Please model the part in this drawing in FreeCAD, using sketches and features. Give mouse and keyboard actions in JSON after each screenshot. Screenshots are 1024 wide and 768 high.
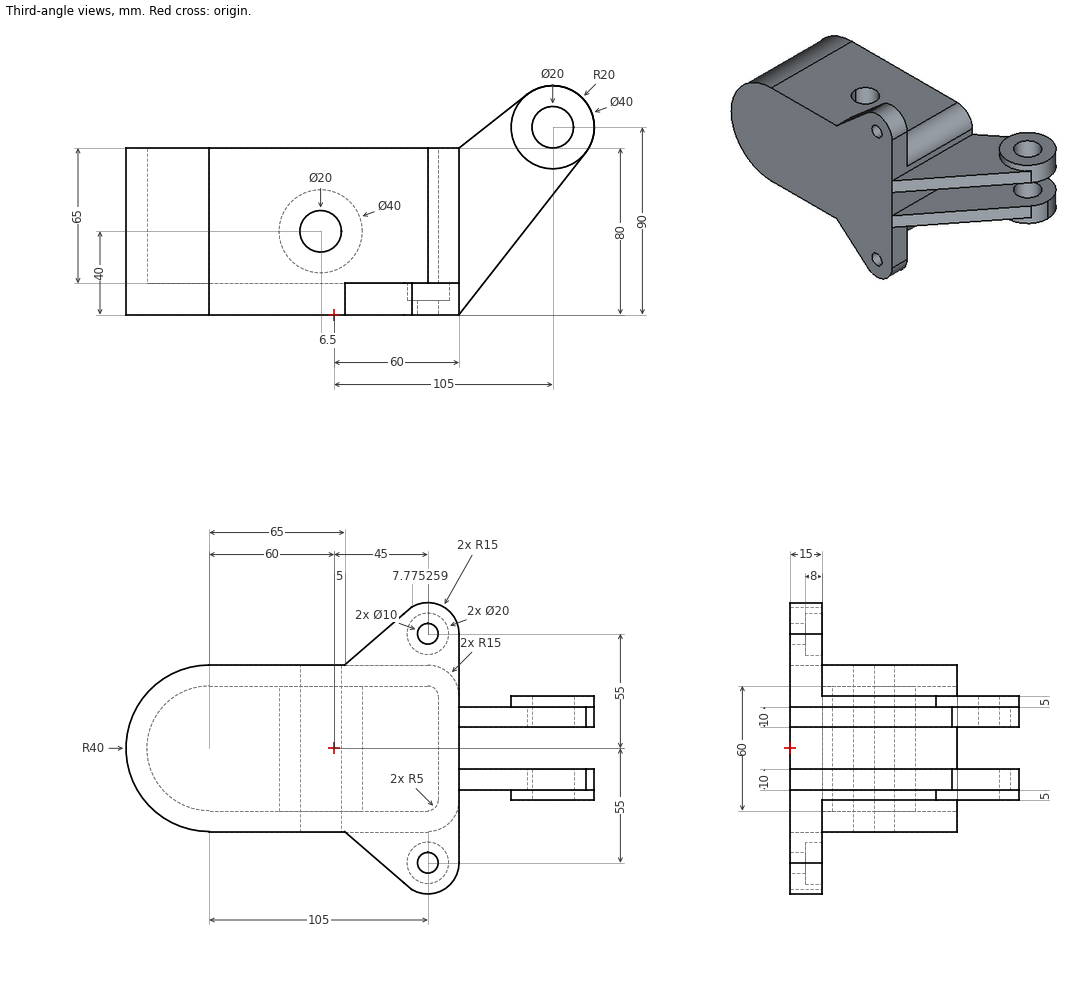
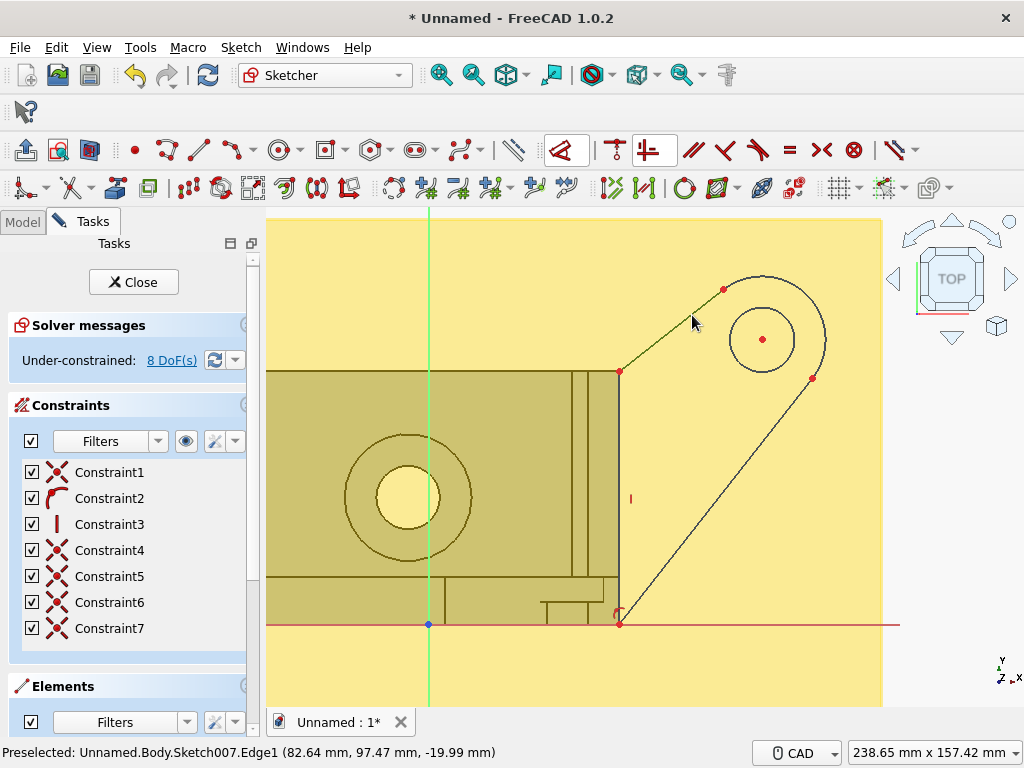
{"action": "left_click", "coordinate": [824, 327]}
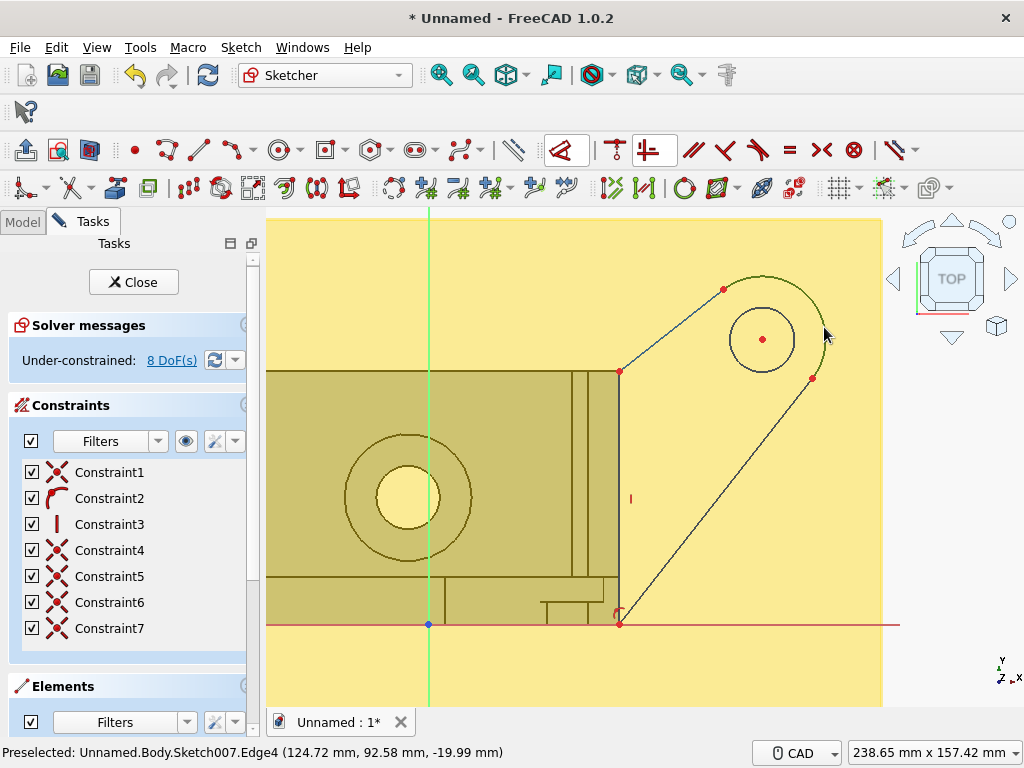
{"action": "left_click", "coordinate": [758, 150]}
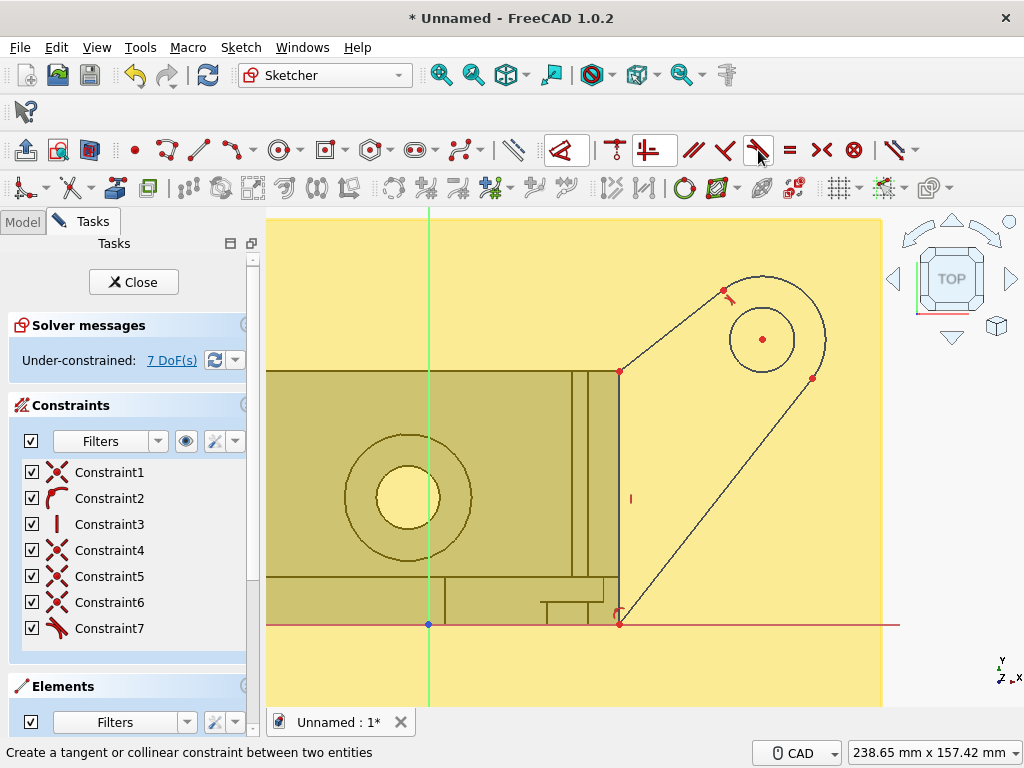
{"action": "left_click", "coordinate": [677, 551]}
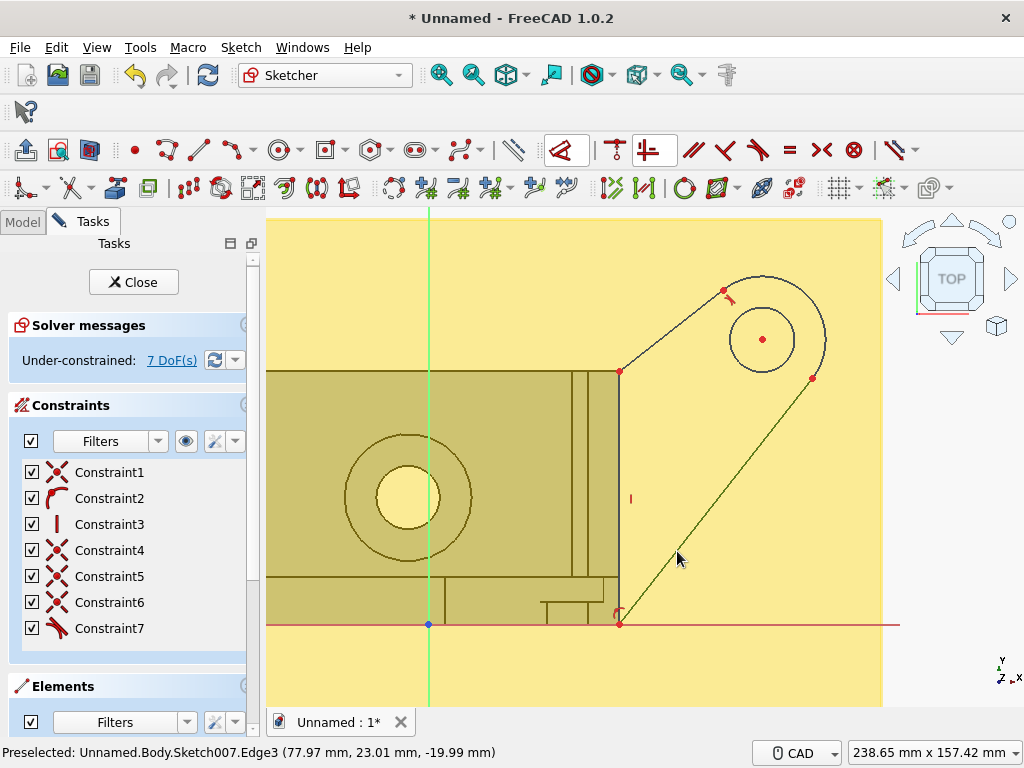
{"action": "left_click", "coordinate": [824, 327]}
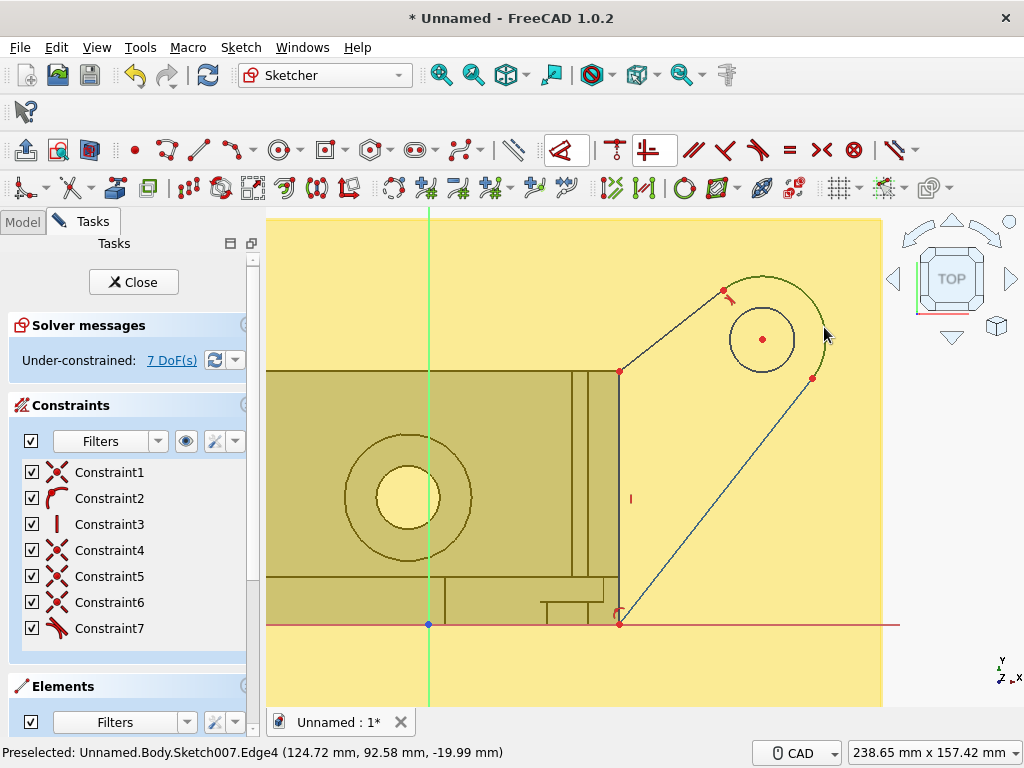
{"action": "left_click", "coordinate": [758, 150]}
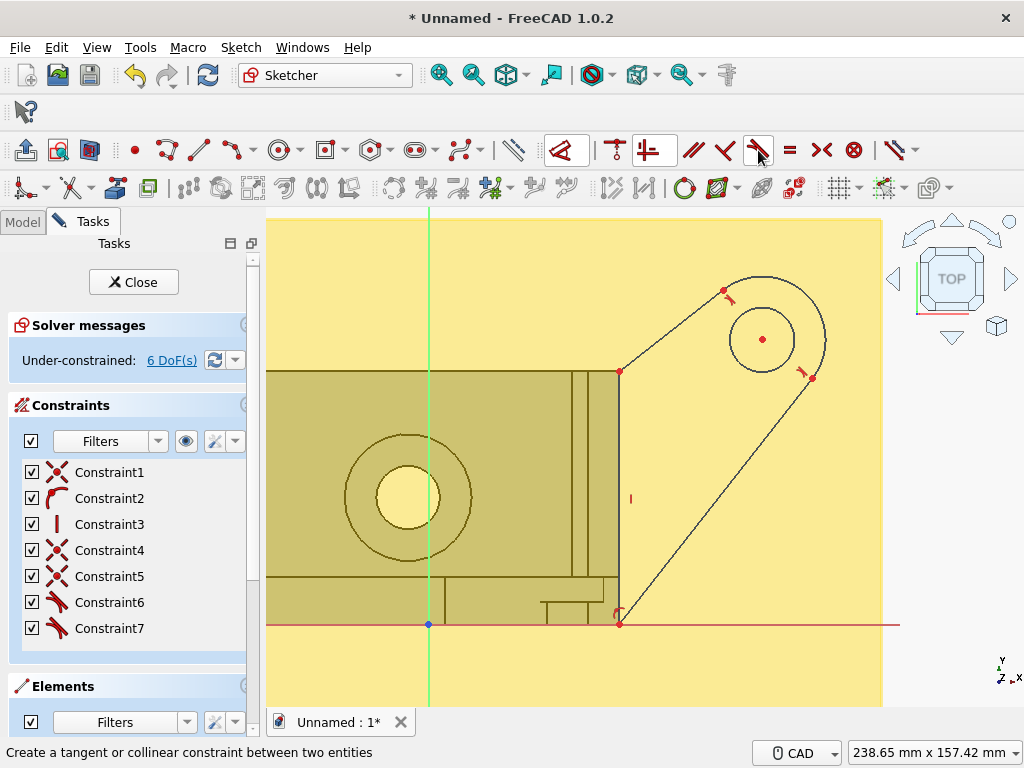
{"action": "left_click", "coordinate": [824, 327]}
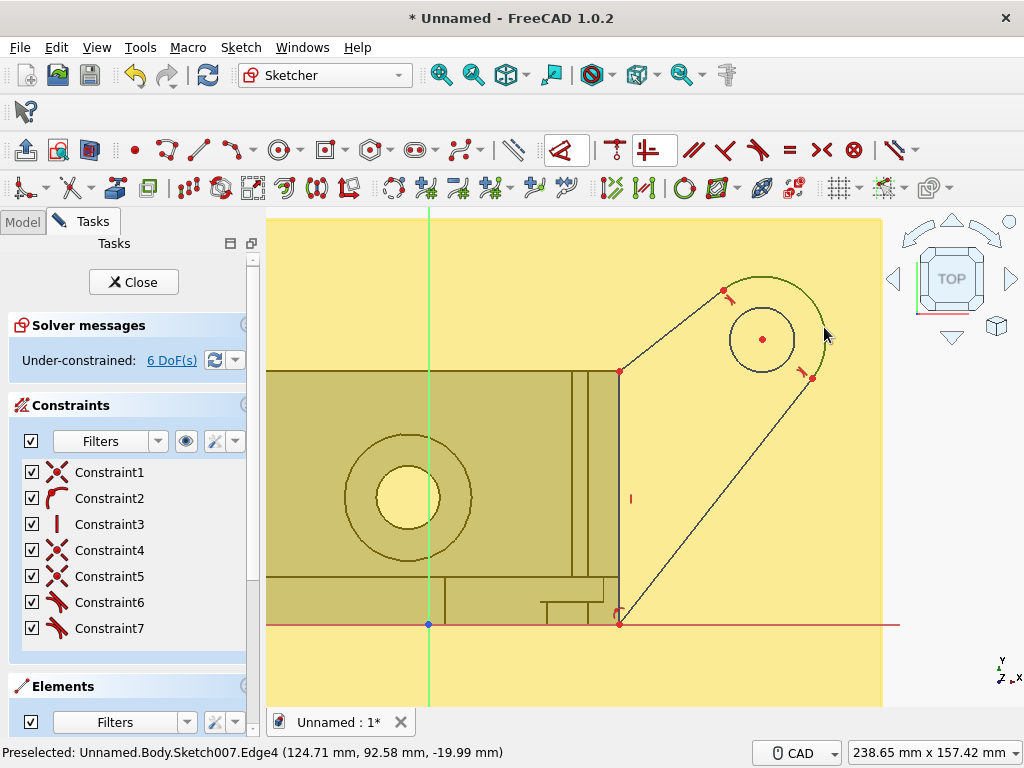
{"action": "left_click", "coordinate": [584, 150]}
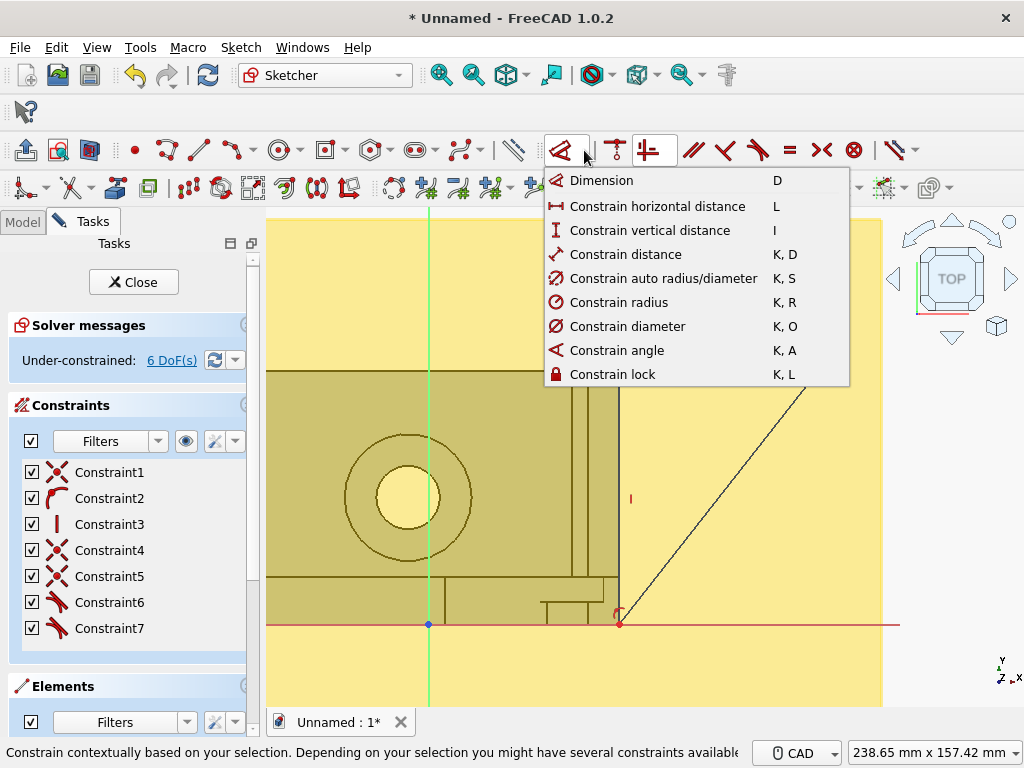
{"action": "left_click", "coordinate": [697, 302]}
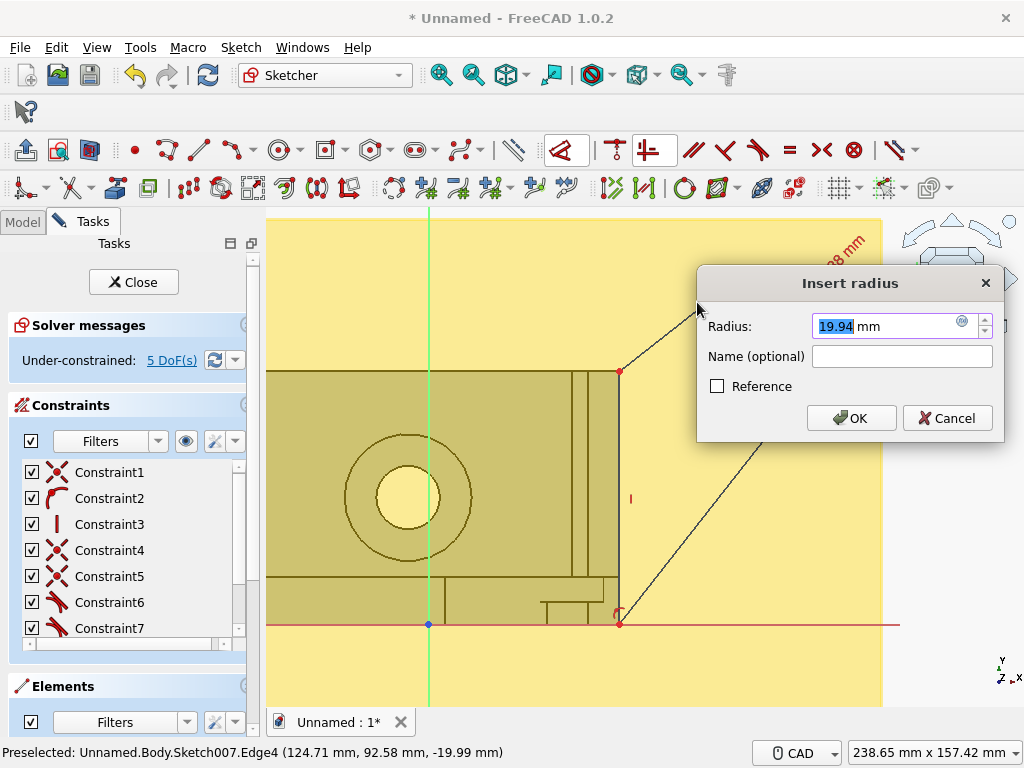
{"action": "type", "text": "20"}
{"action": "key", "text": "Return"}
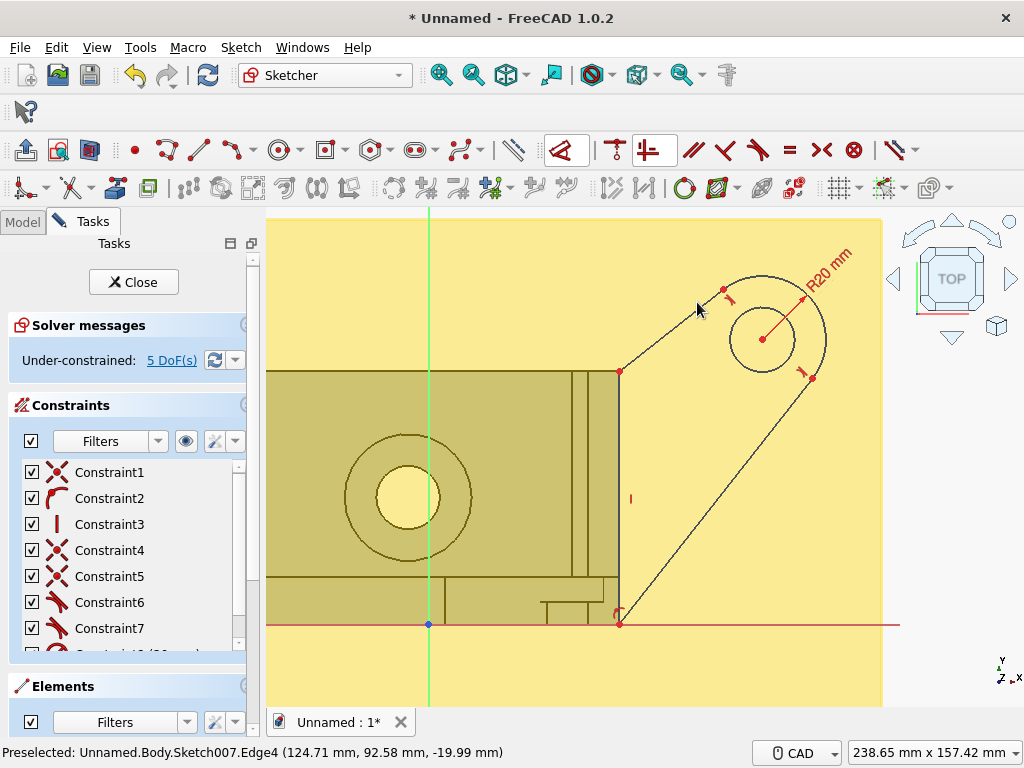
{"action": "left_click", "coordinate": [785, 317]}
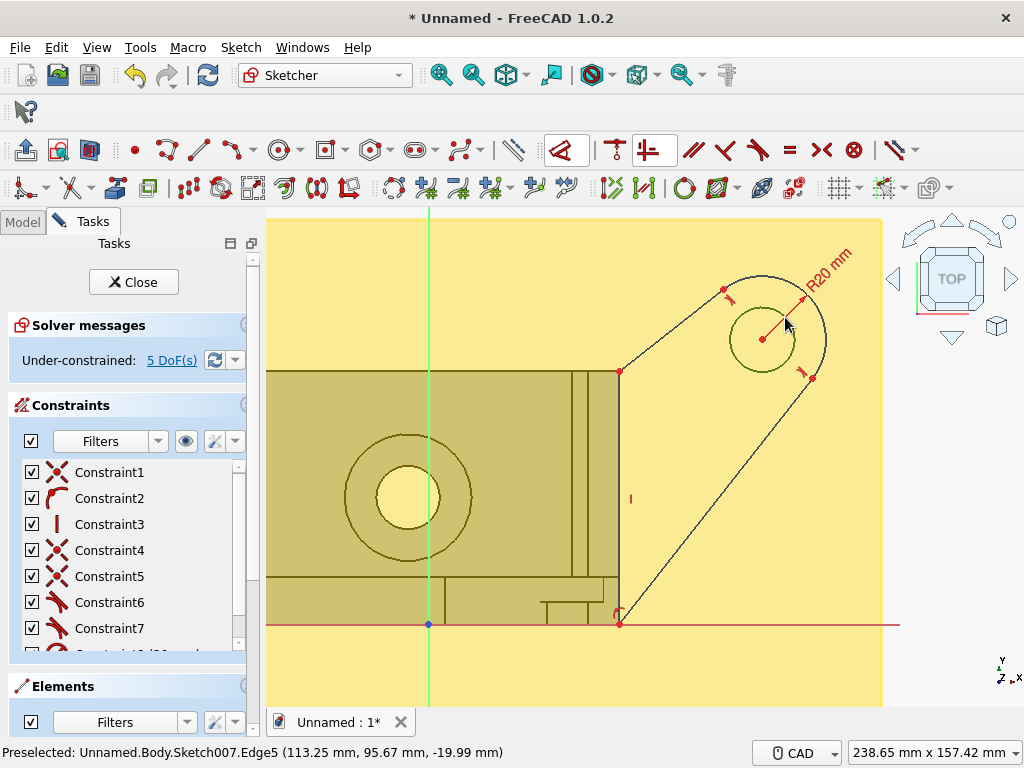
{"action": "left_click", "coordinate": [584, 150]}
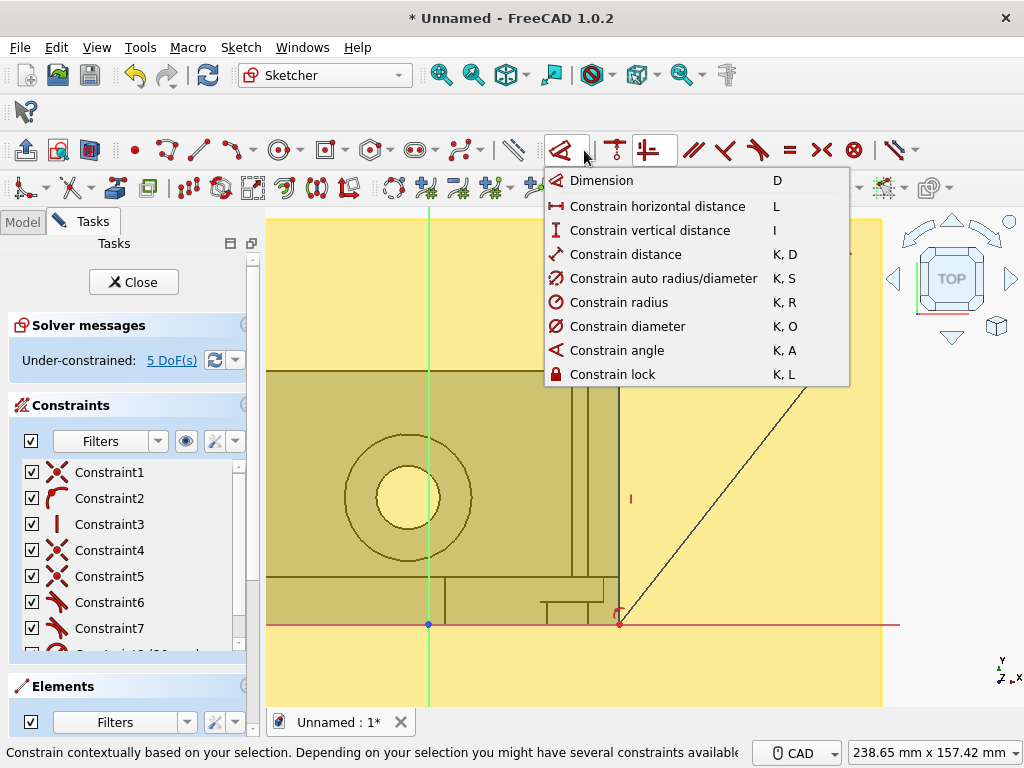
{"action": "left_click", "coordinate": [697, 326]}